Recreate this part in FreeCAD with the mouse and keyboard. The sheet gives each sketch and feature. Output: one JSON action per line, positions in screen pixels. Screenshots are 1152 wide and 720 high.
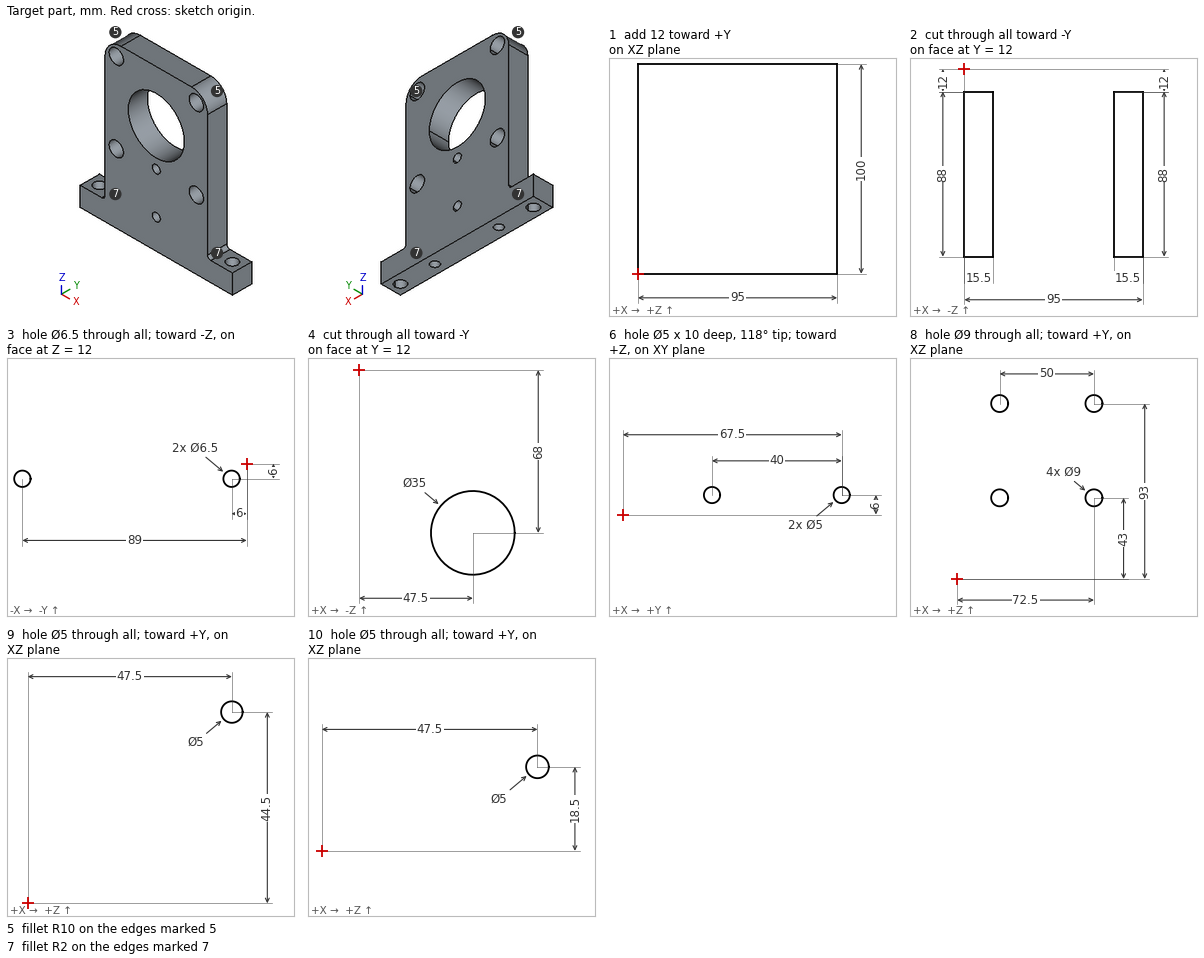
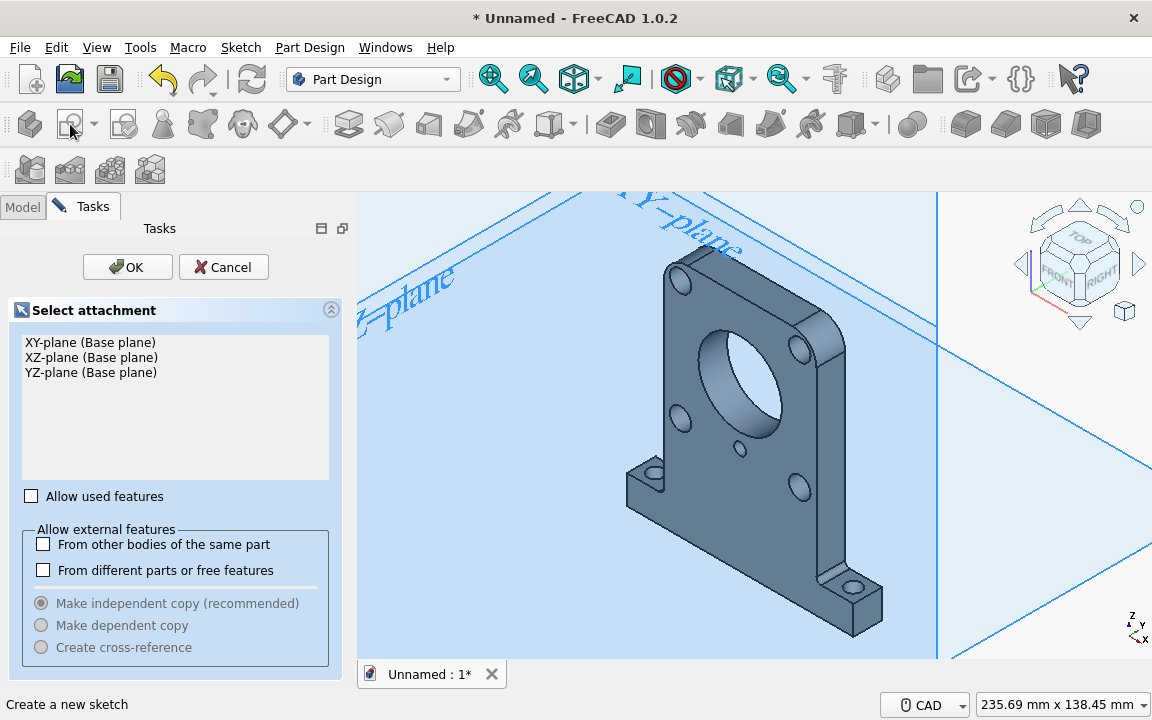
{"action": "left_click", "coordinate": [82, 358]}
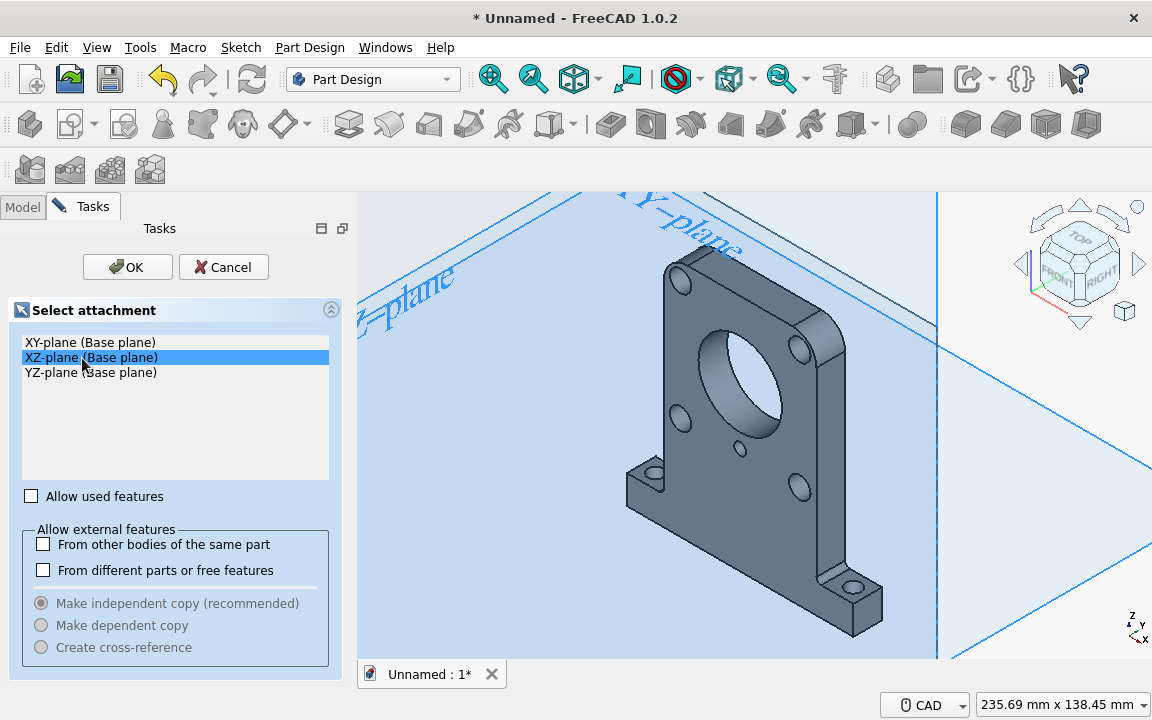
{"action": "left_click", "coordinate": [128, 267]}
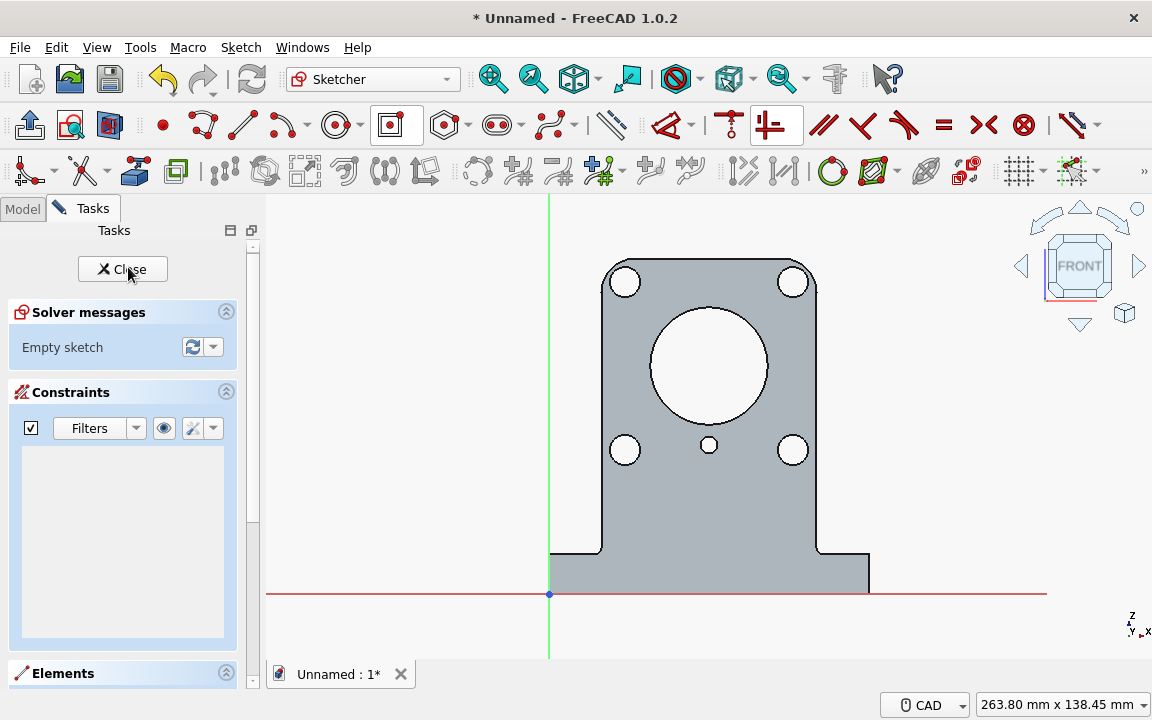
{"action": "scroll", "coordinate": [713, 539], "scroll_direction": "up", "scroll_amount": 14}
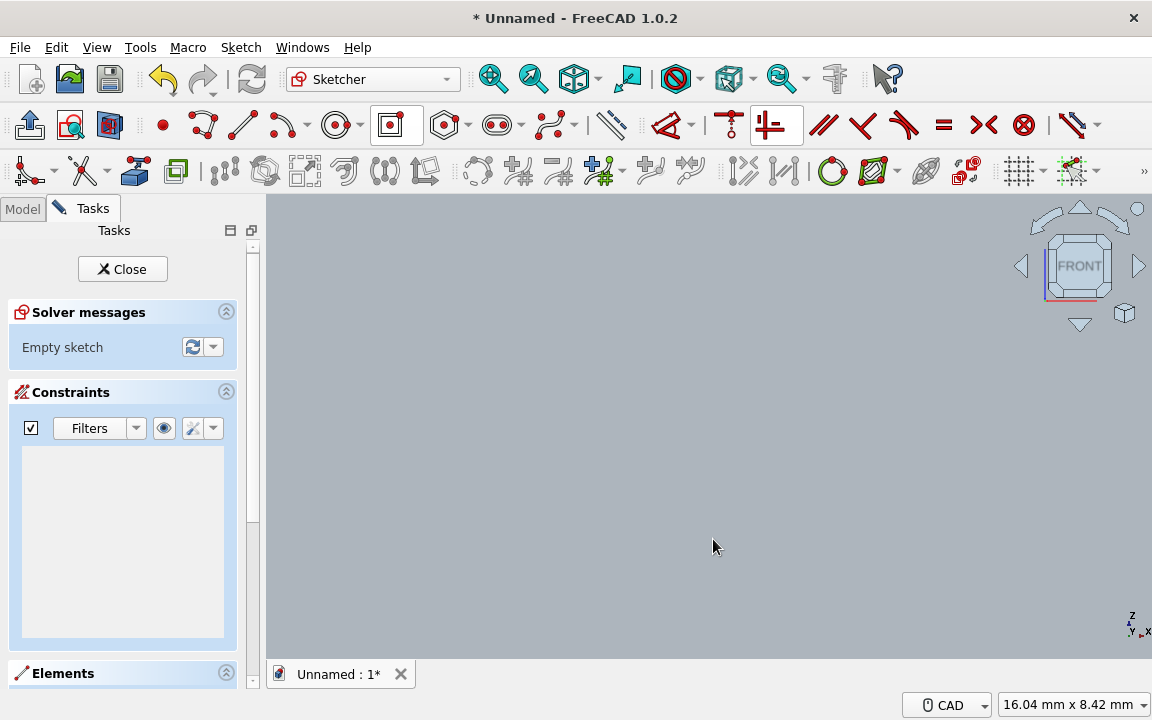
{"action": "left_click", "coordinate": [336, 126]}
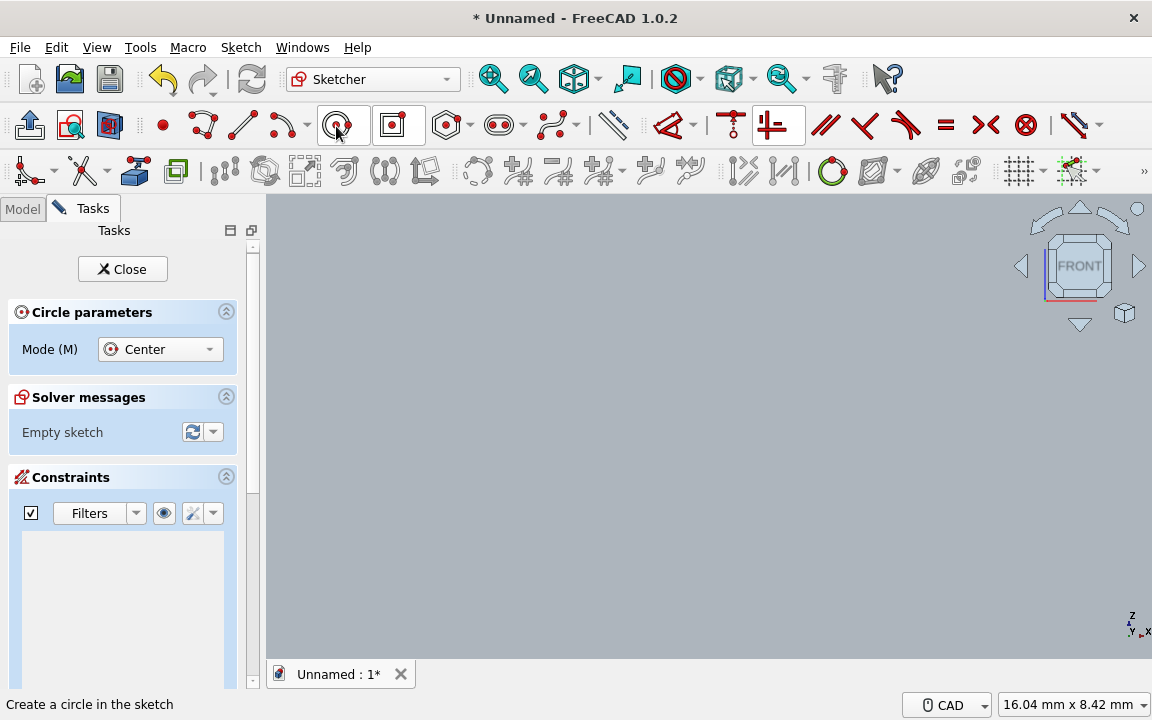
{"action": "left_click", "coordinate": [639, 417]}
{"action": "left_click", "coordinate": [737, 320]}
{"action": "key", "text": "Escape"}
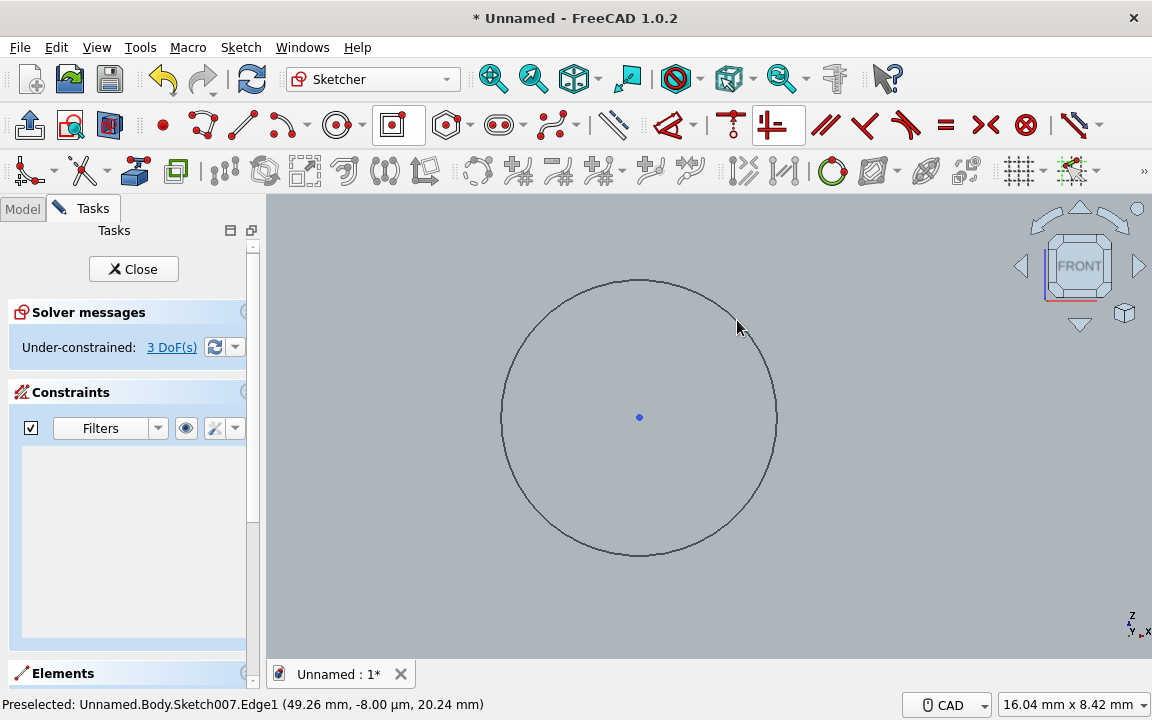
{"action": "left_click", "coordinate": [668, 126]}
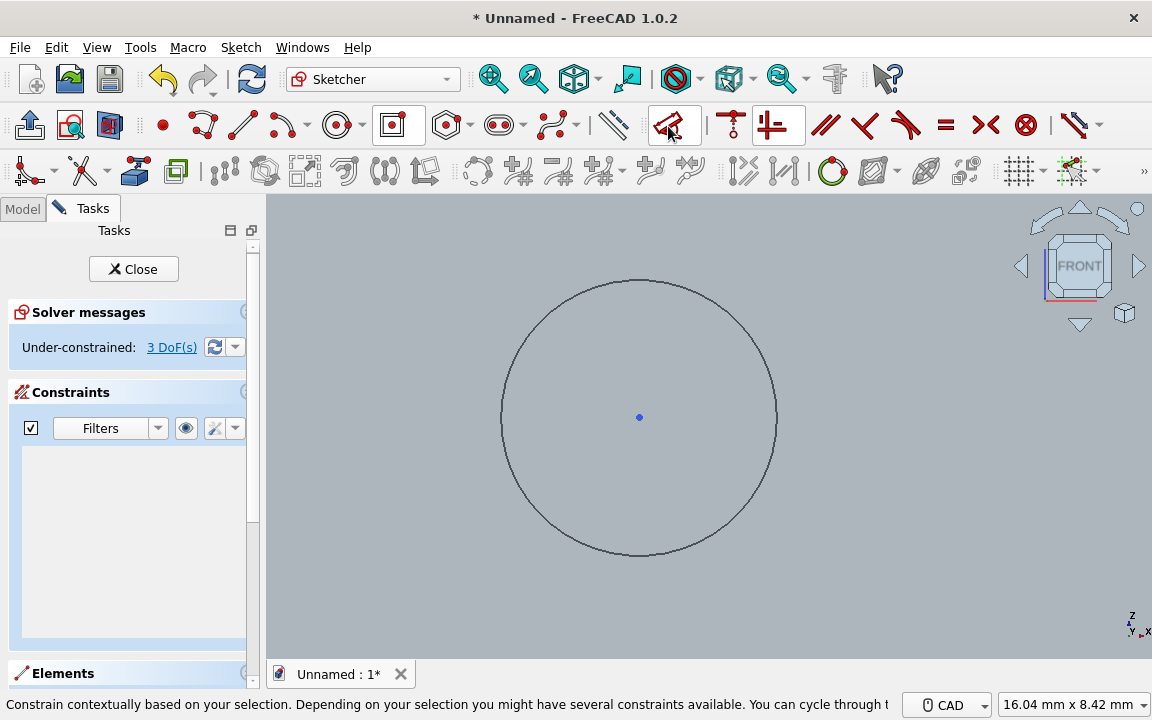
{"action": "left_click", "coordinate": [736, 320]}
{"action": "left_click", "coordinate": [759, 297]}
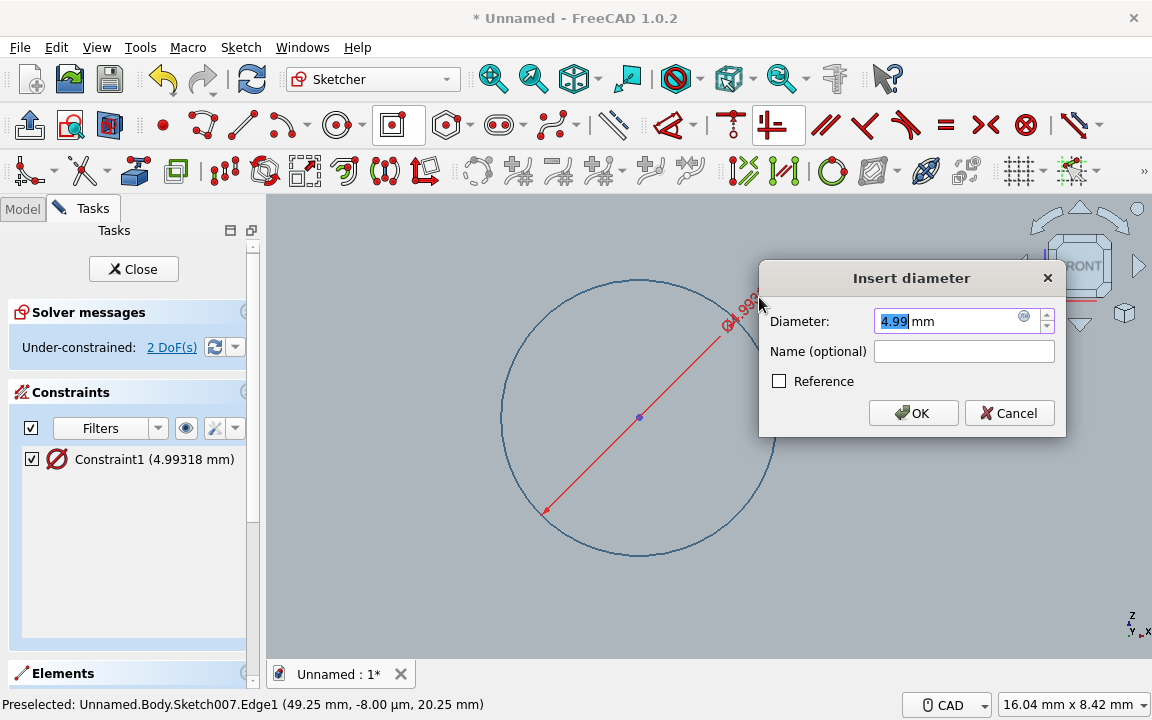
{"action": "type", "text": "5"}
{"action": "key", "text": "Return"}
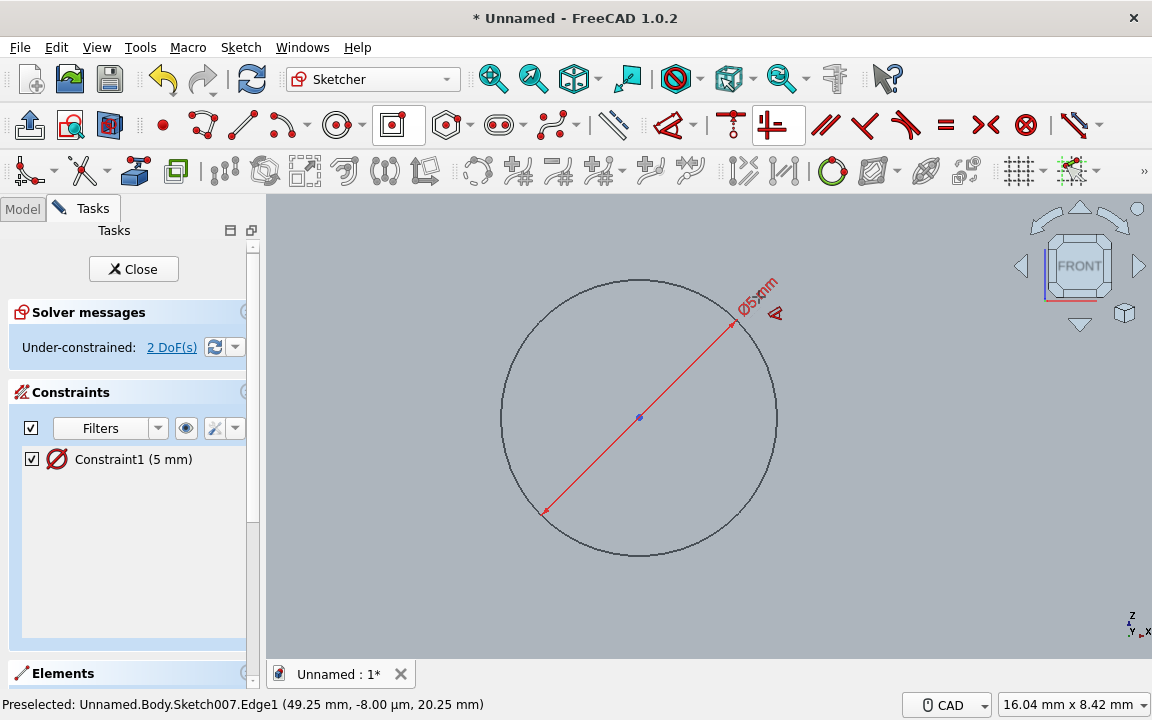
{"action": "left_click", "coordinate": [639, 418]}
{"action": "left_click", "coordinate": [467, 384]}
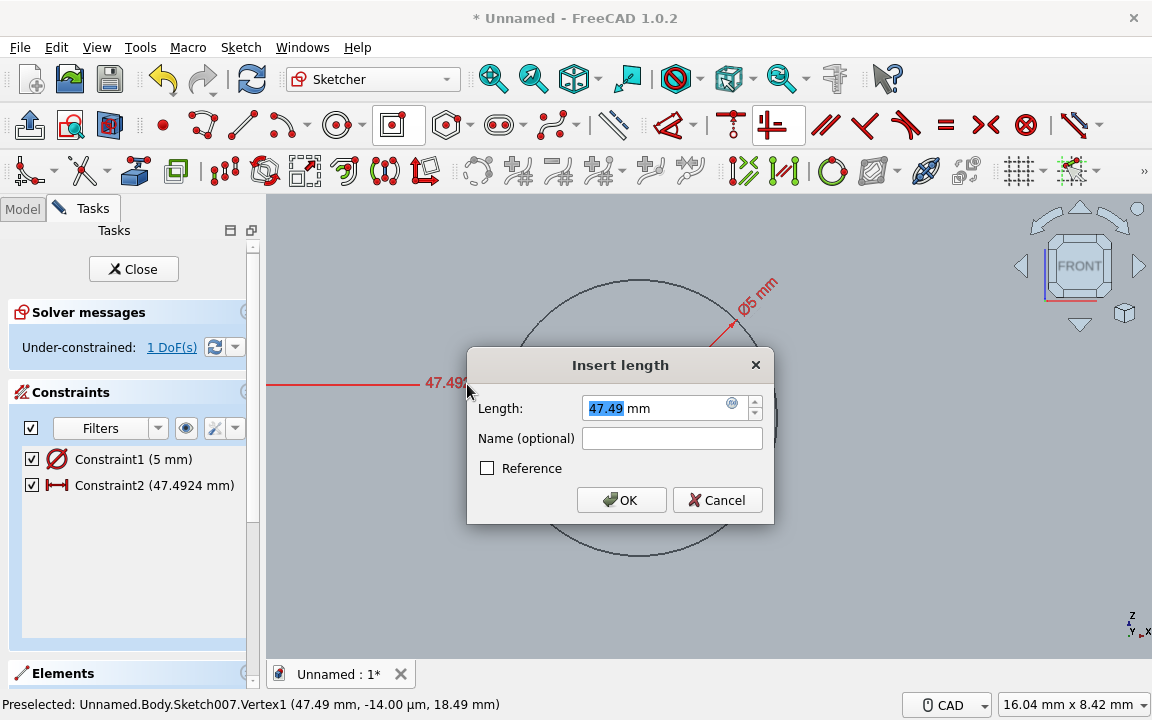
{"action": "type", "text": "47.5"}
{"action": "key", "text": "Return"}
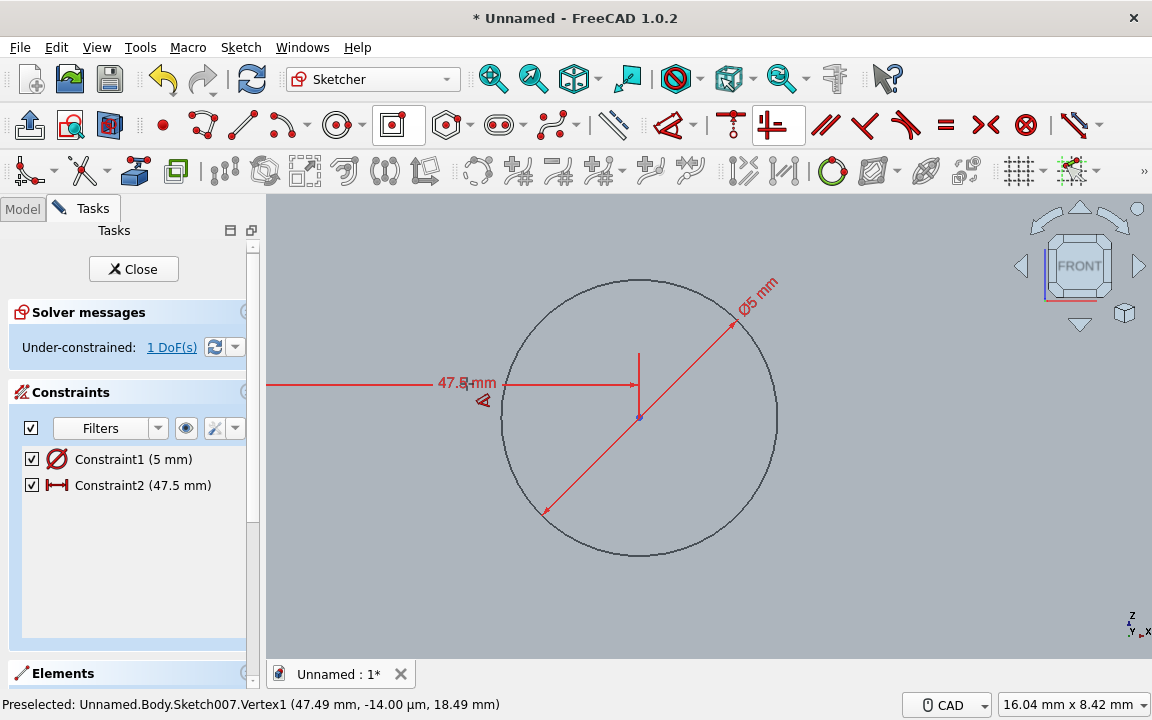
{"action": "left_click", "coordinate": [639, 418]}
{"action": "left_click", "coordinate": [673, 525]}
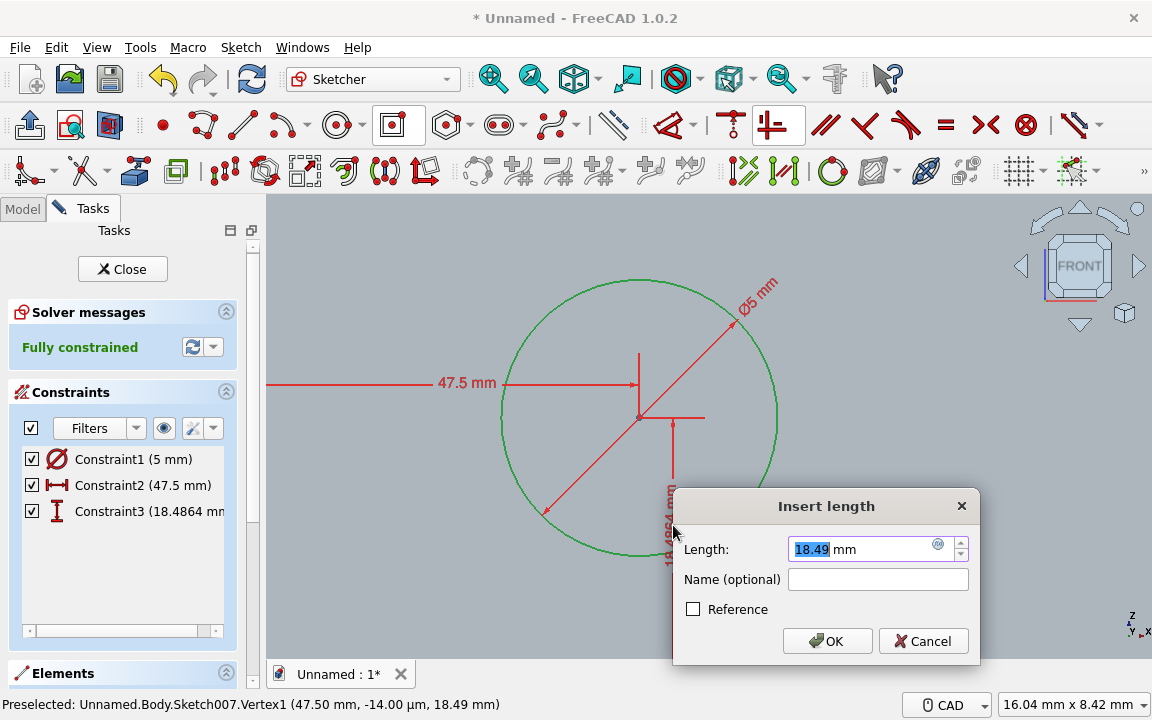
{"action": "type", "text": "18.5"}
{"action": "key", "text": "Return"}
{"action": "key", "text": "Escape"}